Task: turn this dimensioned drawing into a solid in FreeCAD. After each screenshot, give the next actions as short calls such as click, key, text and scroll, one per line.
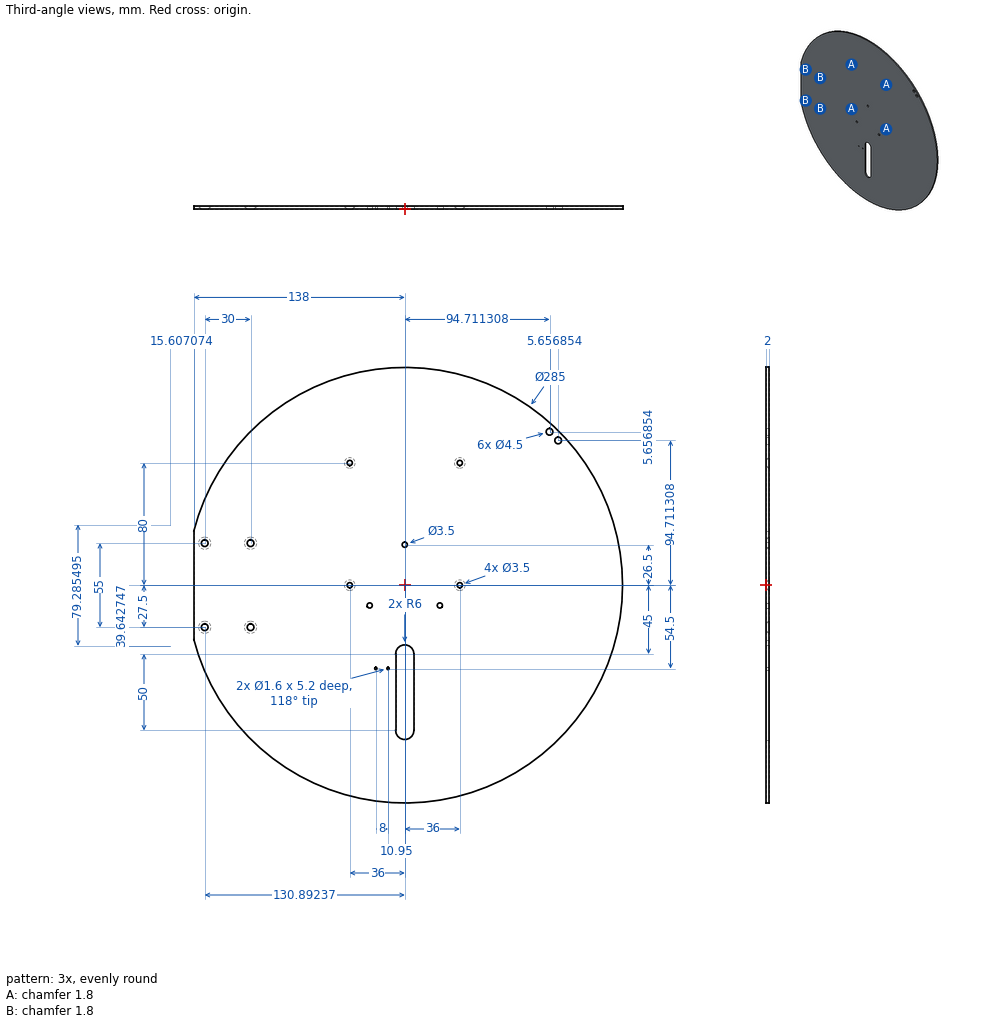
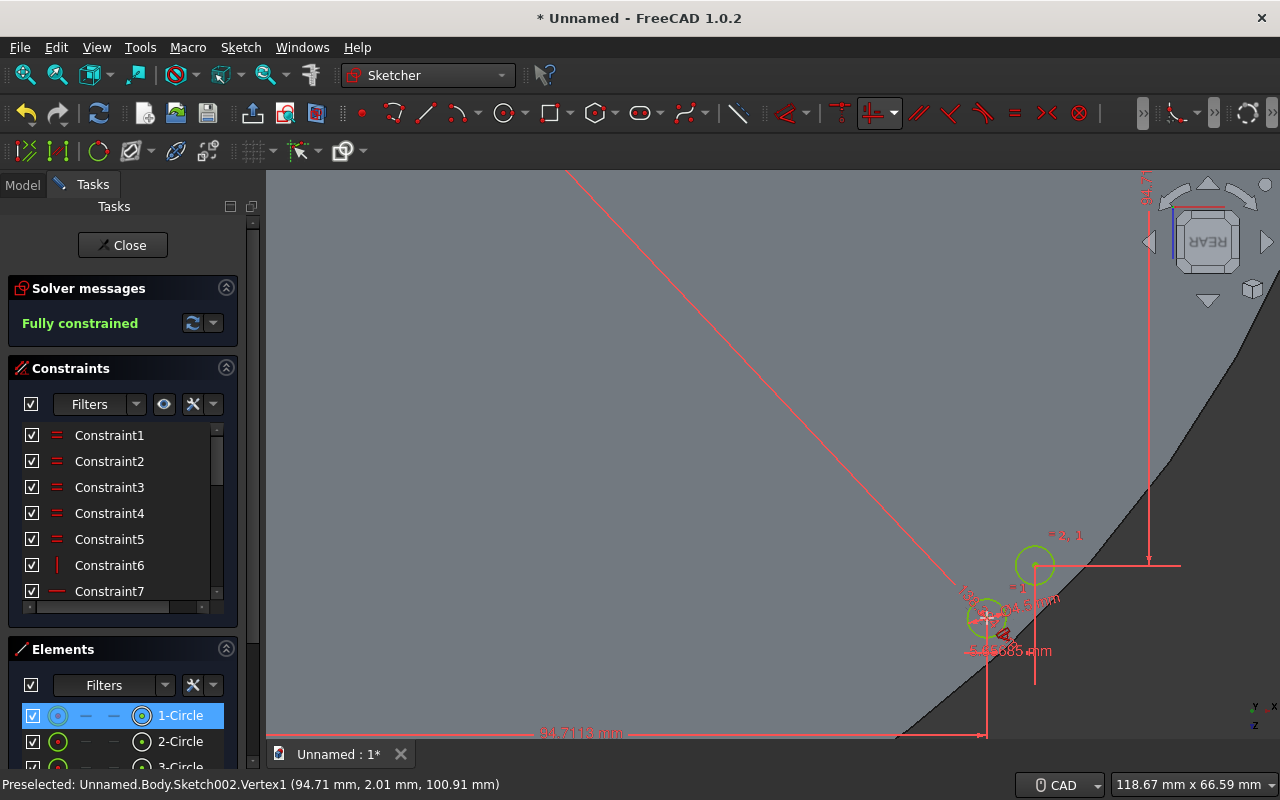
click(1035, 566)
click(1069, 580)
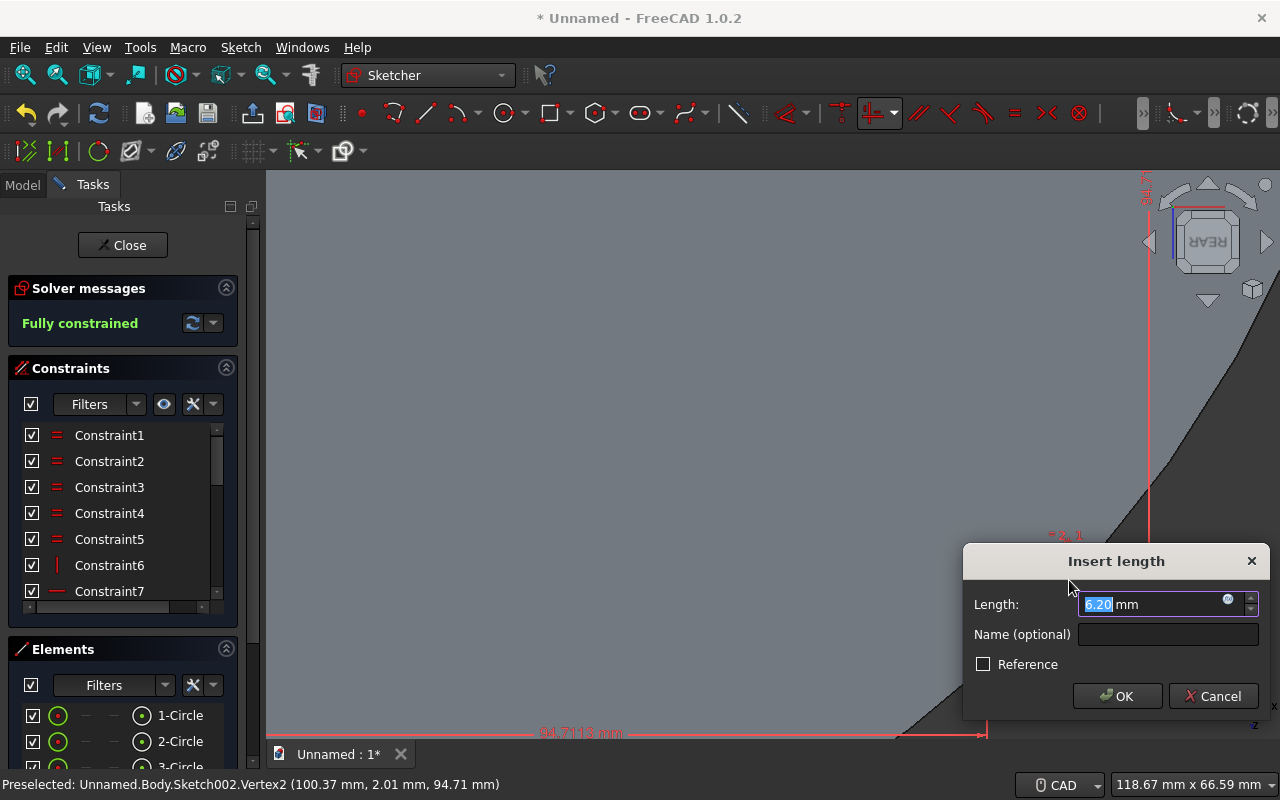
text(5.656854)
key(Return)
key(Escape)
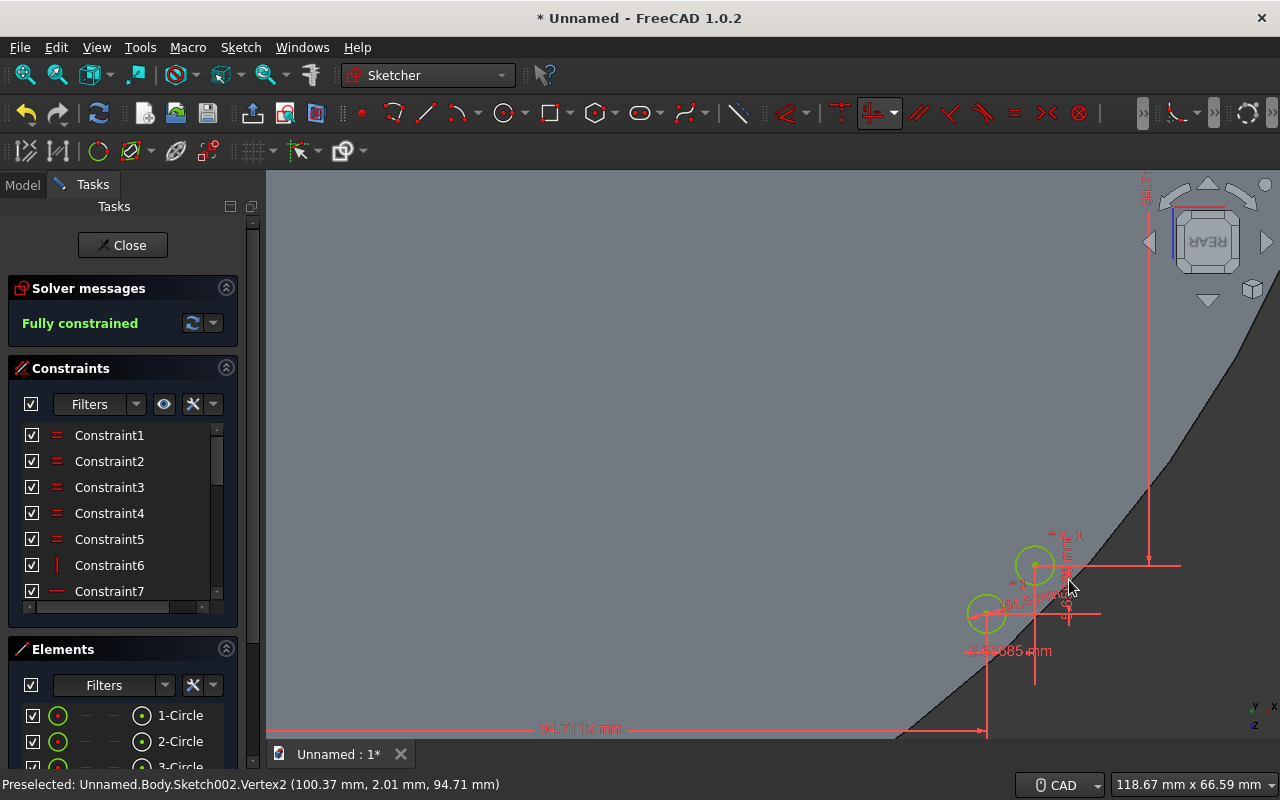
click(123, 245)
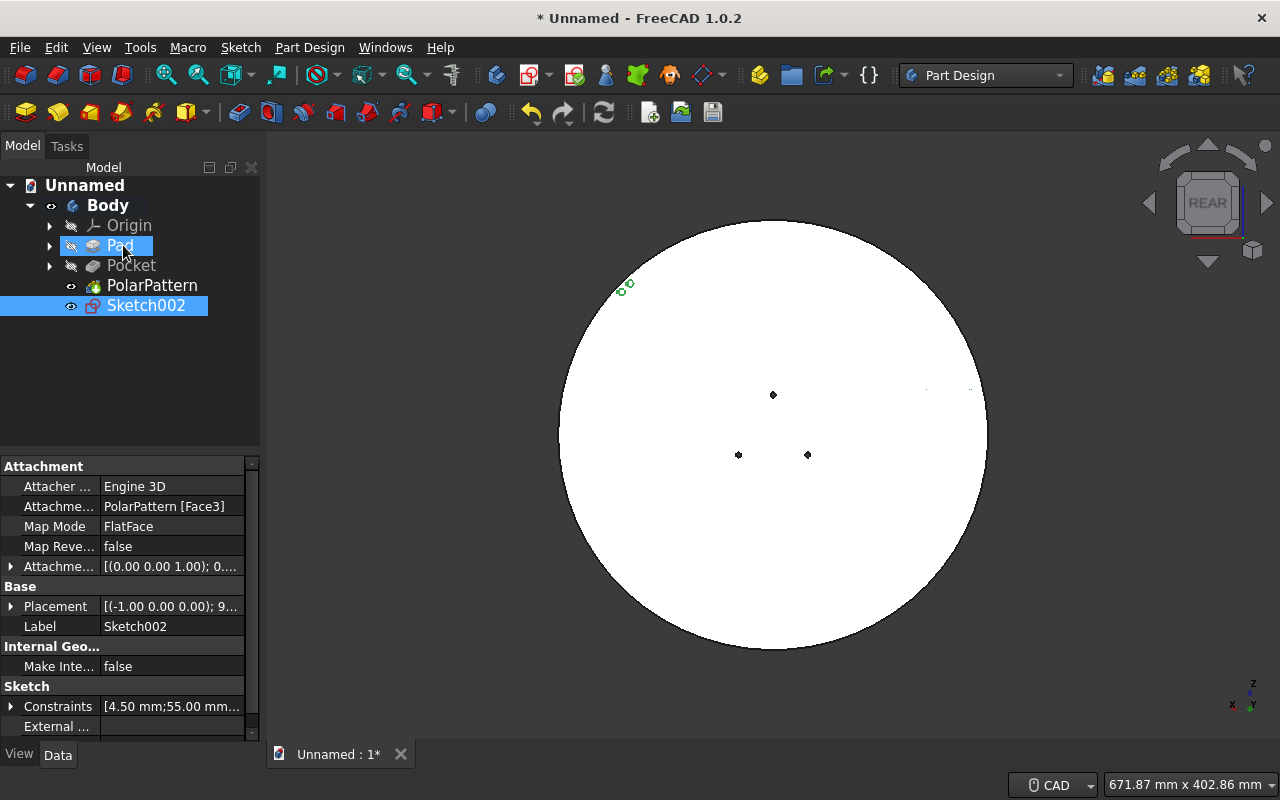
click(240, 112)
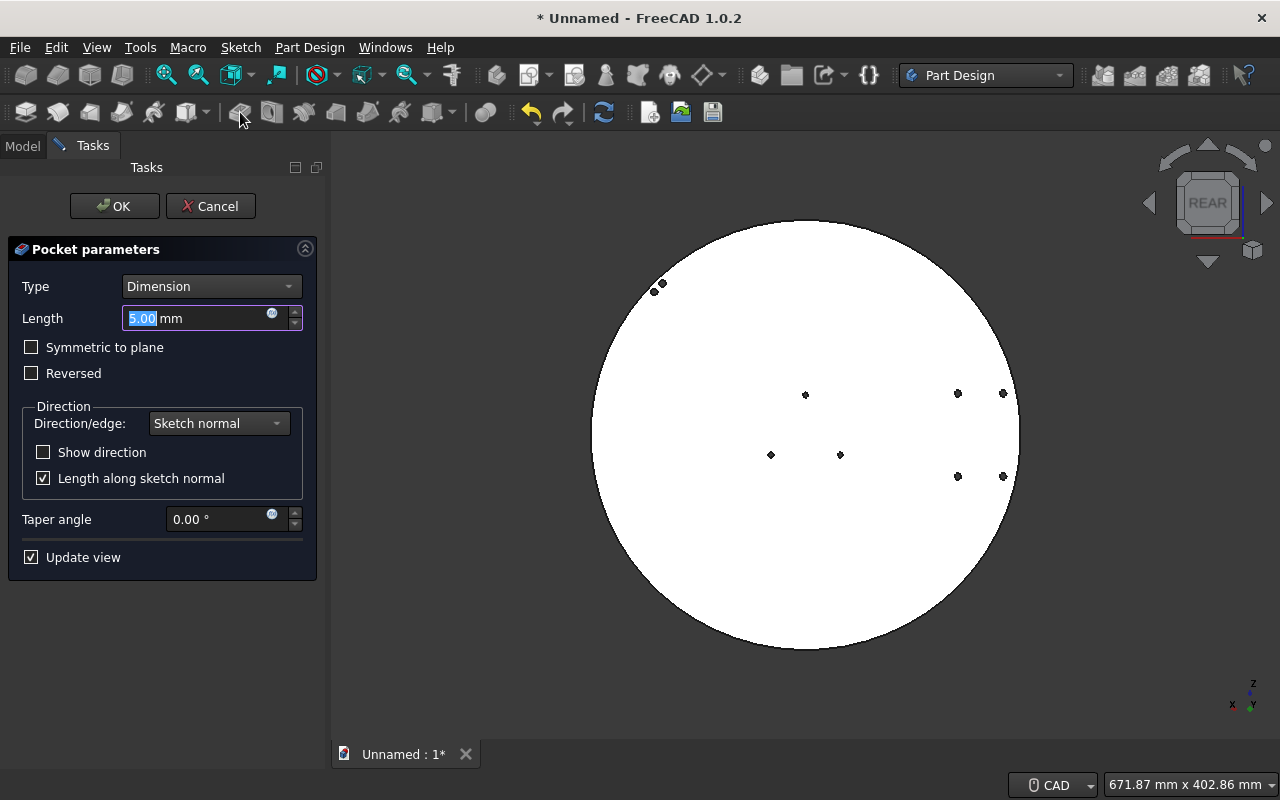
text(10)
key(Tab)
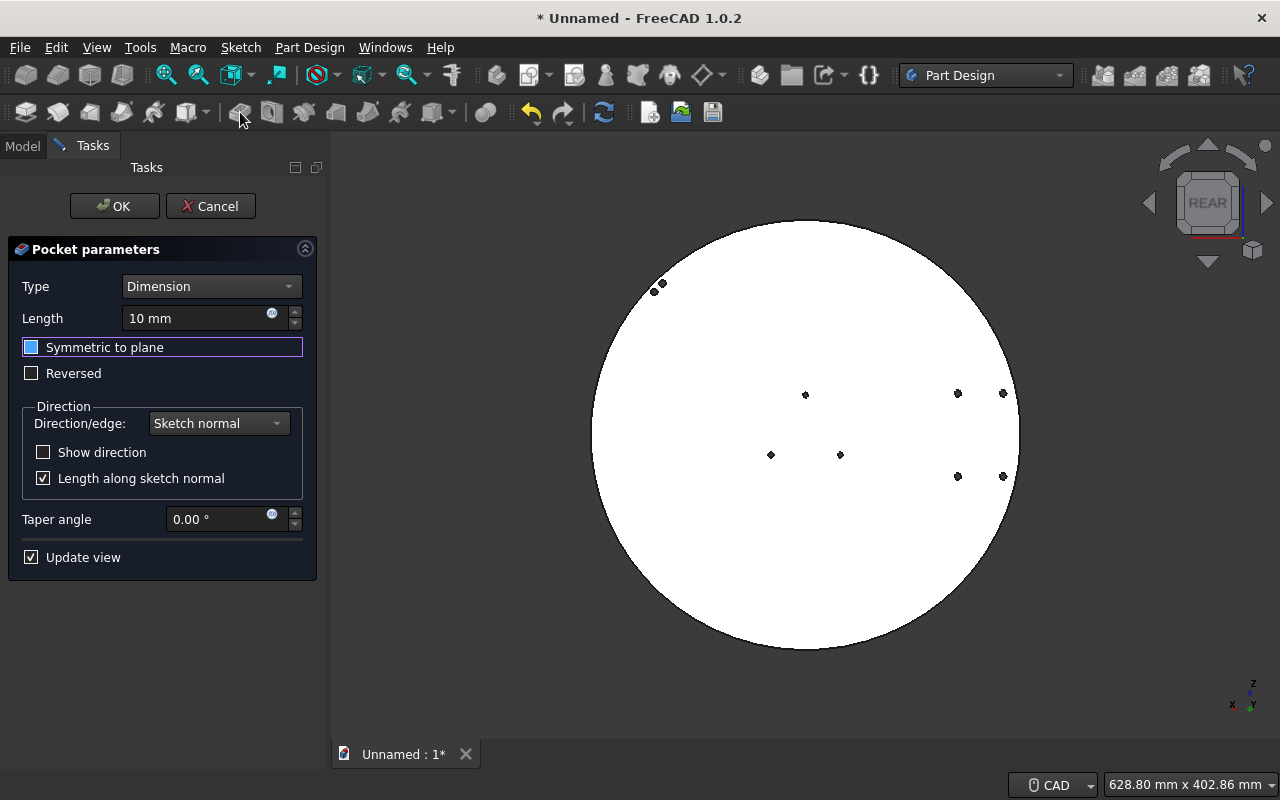
click(115, 206)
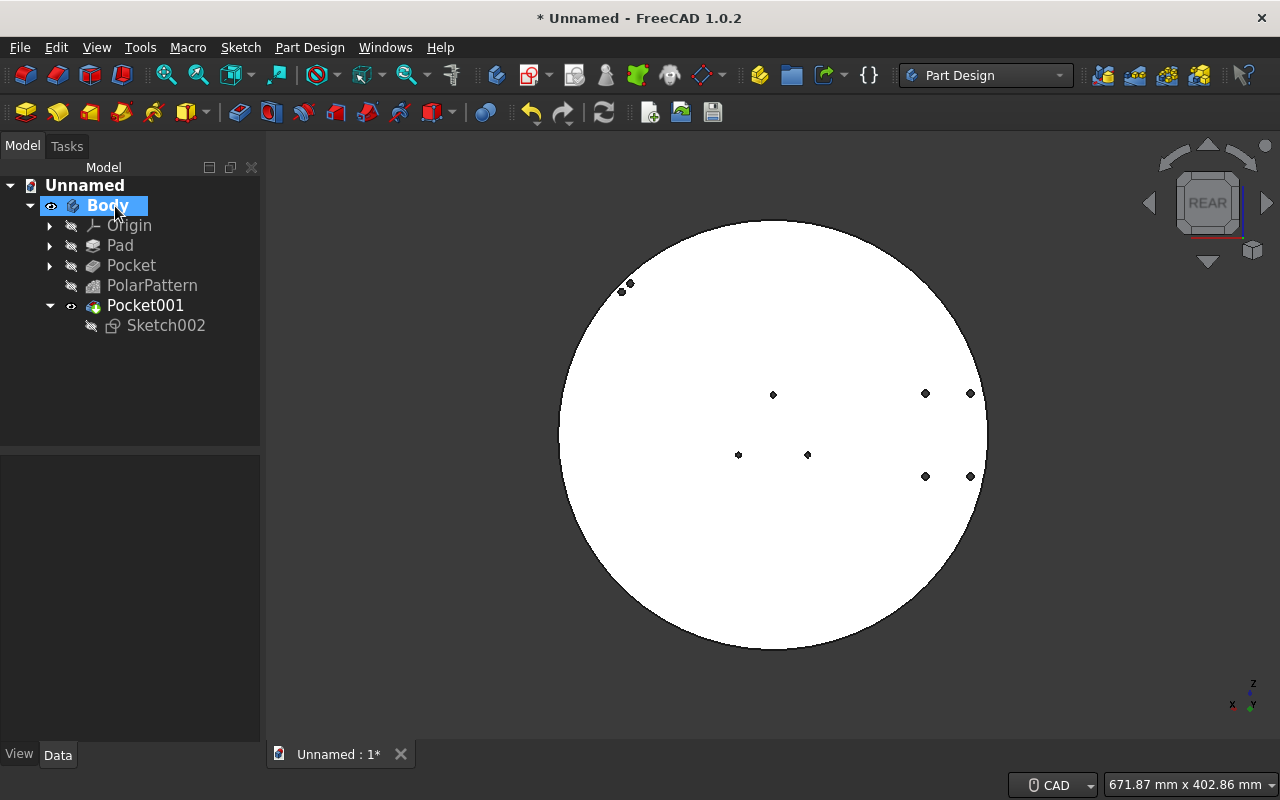
click(773, 557)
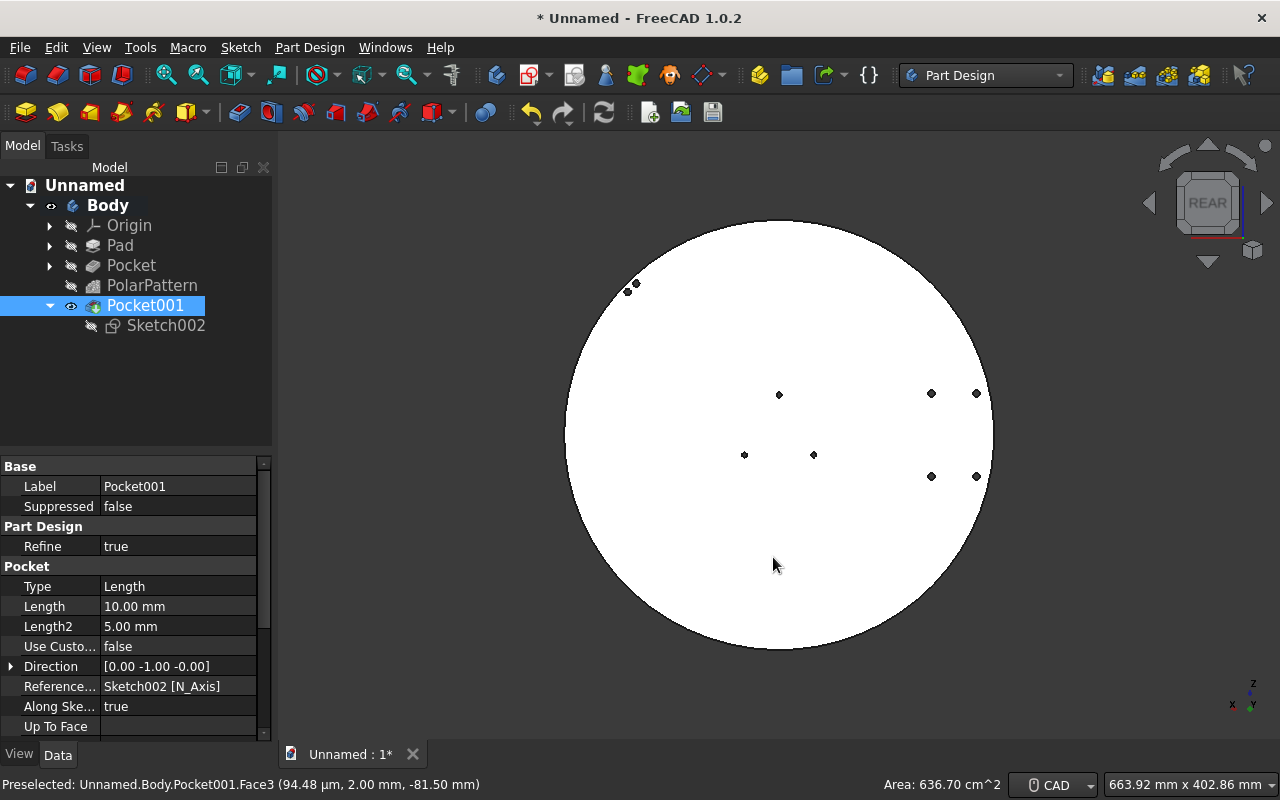
click(530, 76)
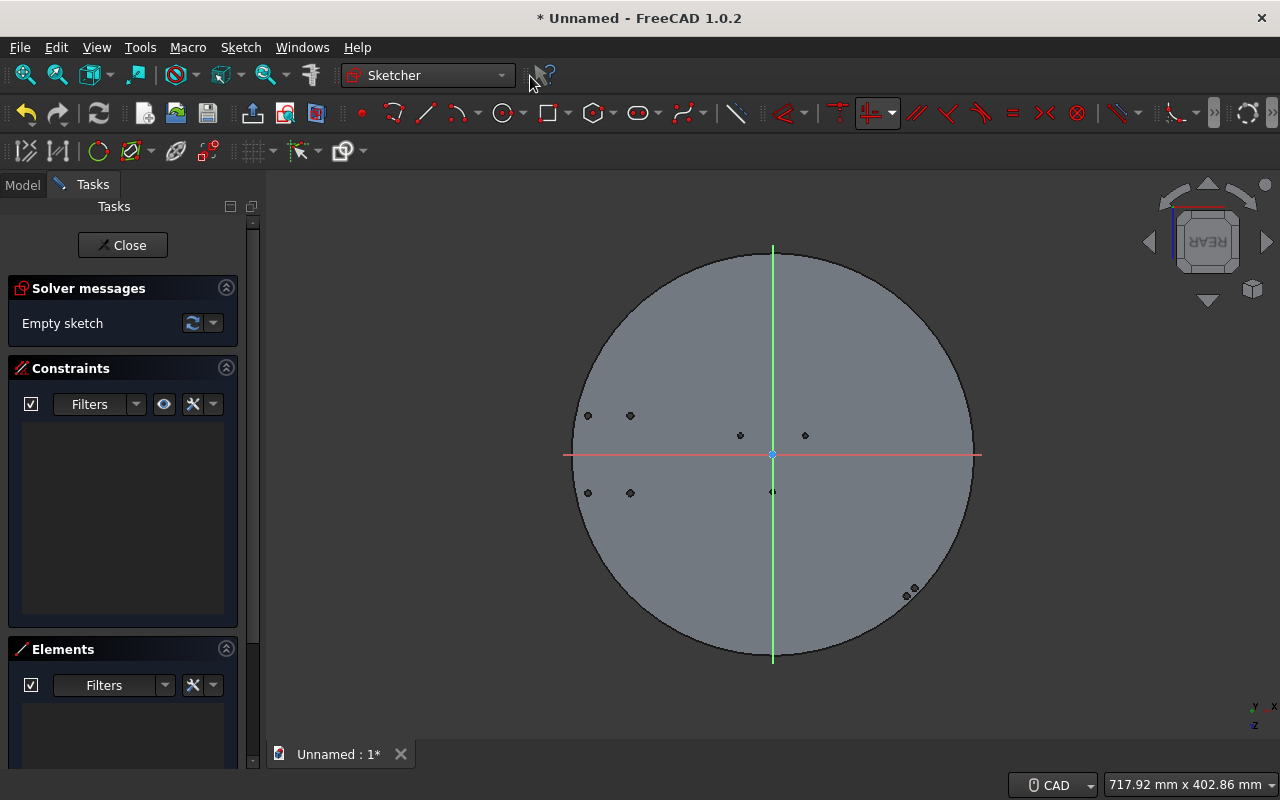
scroll(813, 342, up, 5)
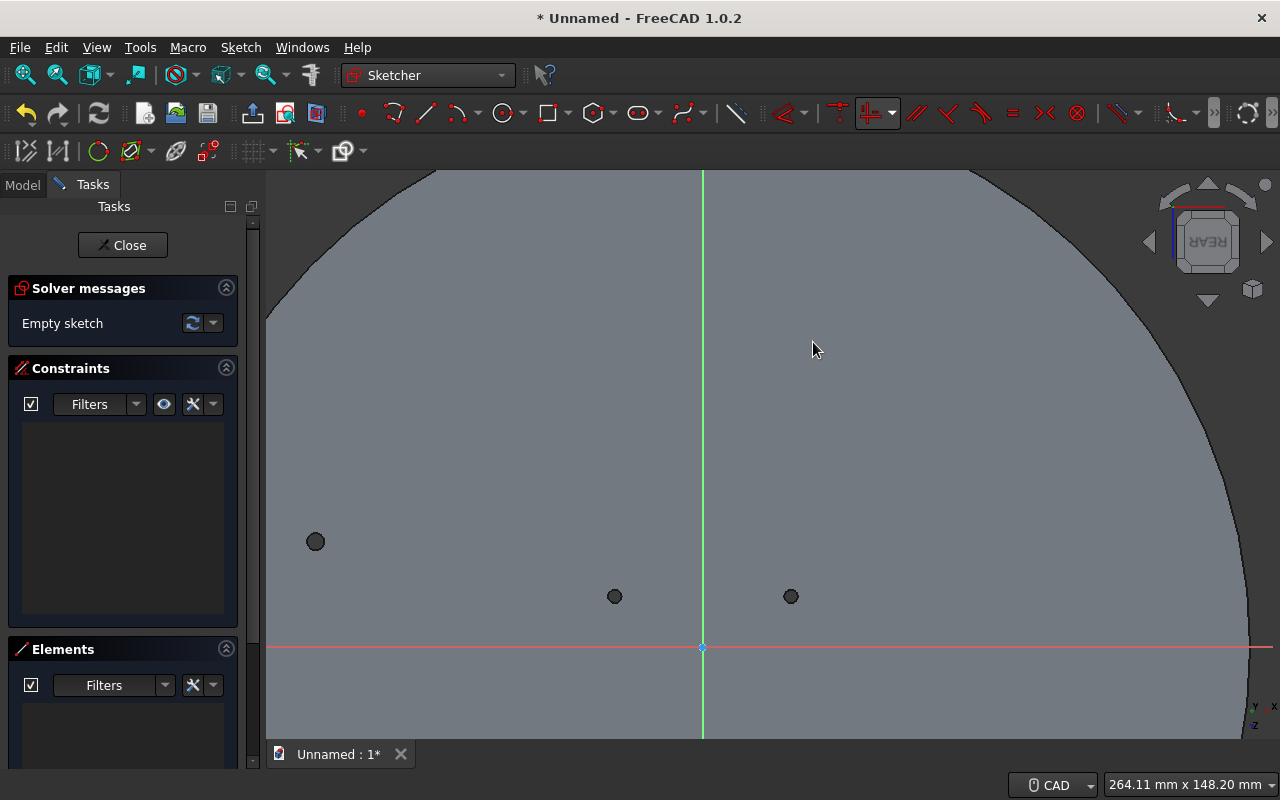
click(638, 114)